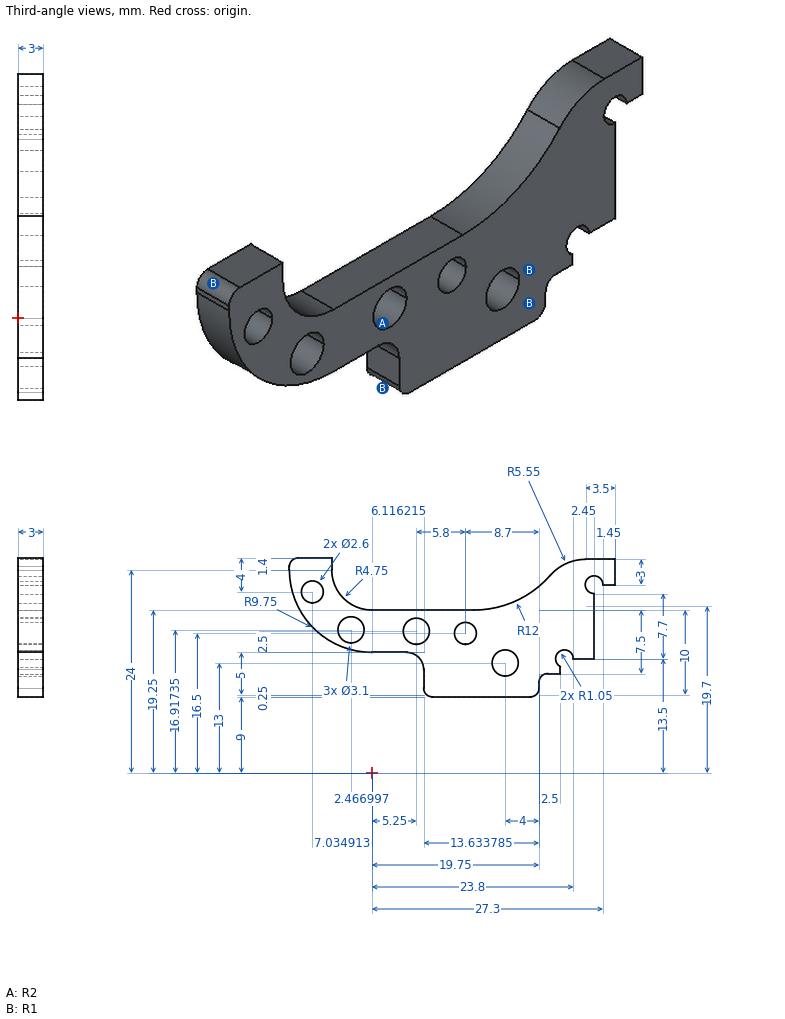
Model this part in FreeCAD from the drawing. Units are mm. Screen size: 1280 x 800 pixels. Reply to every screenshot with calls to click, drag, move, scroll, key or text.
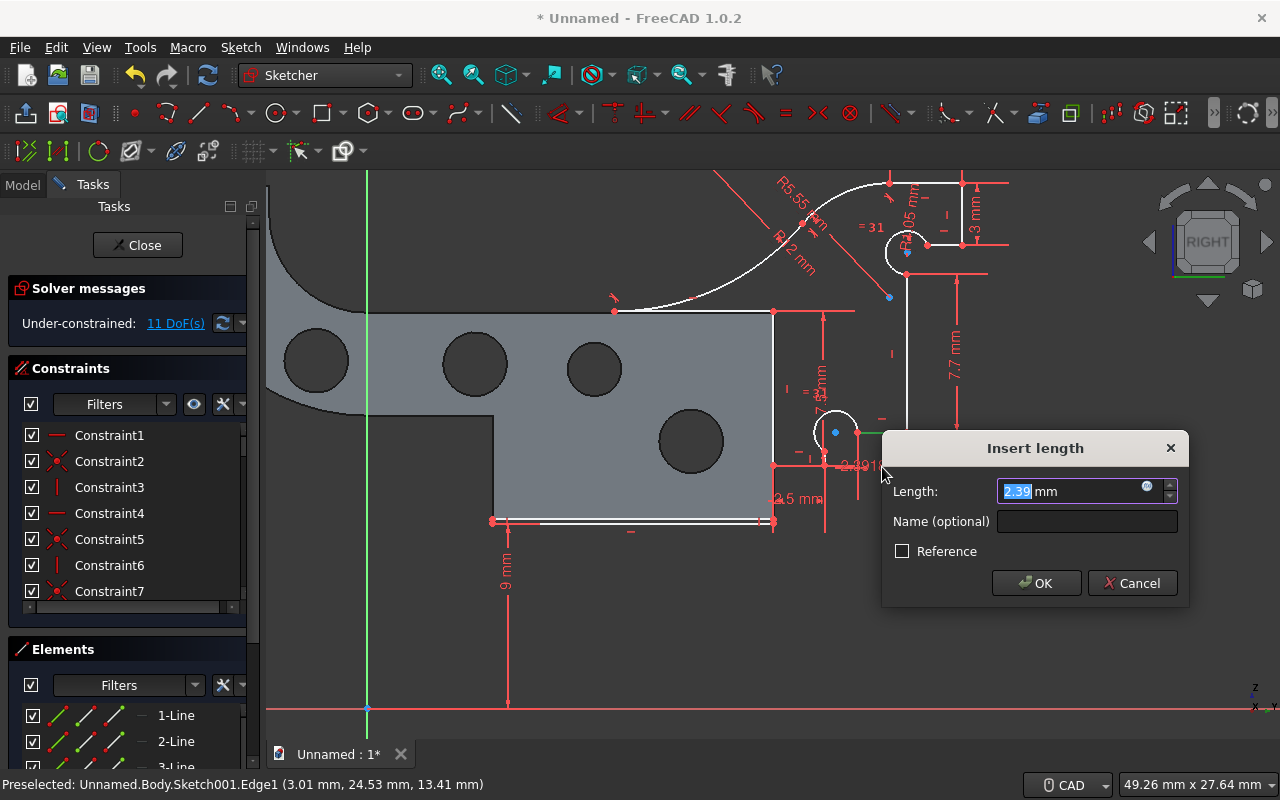
text(2.45)
key(Return)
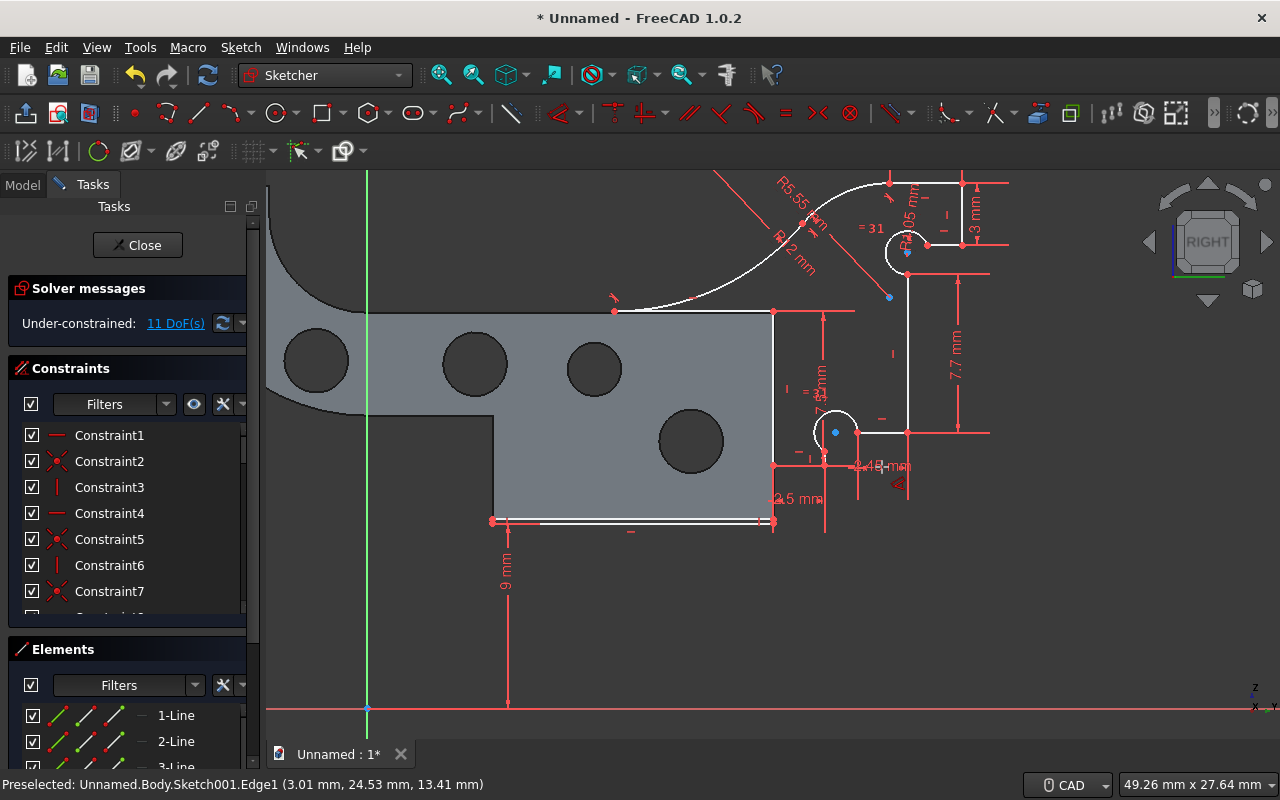
scroll(938, 245, up, 2)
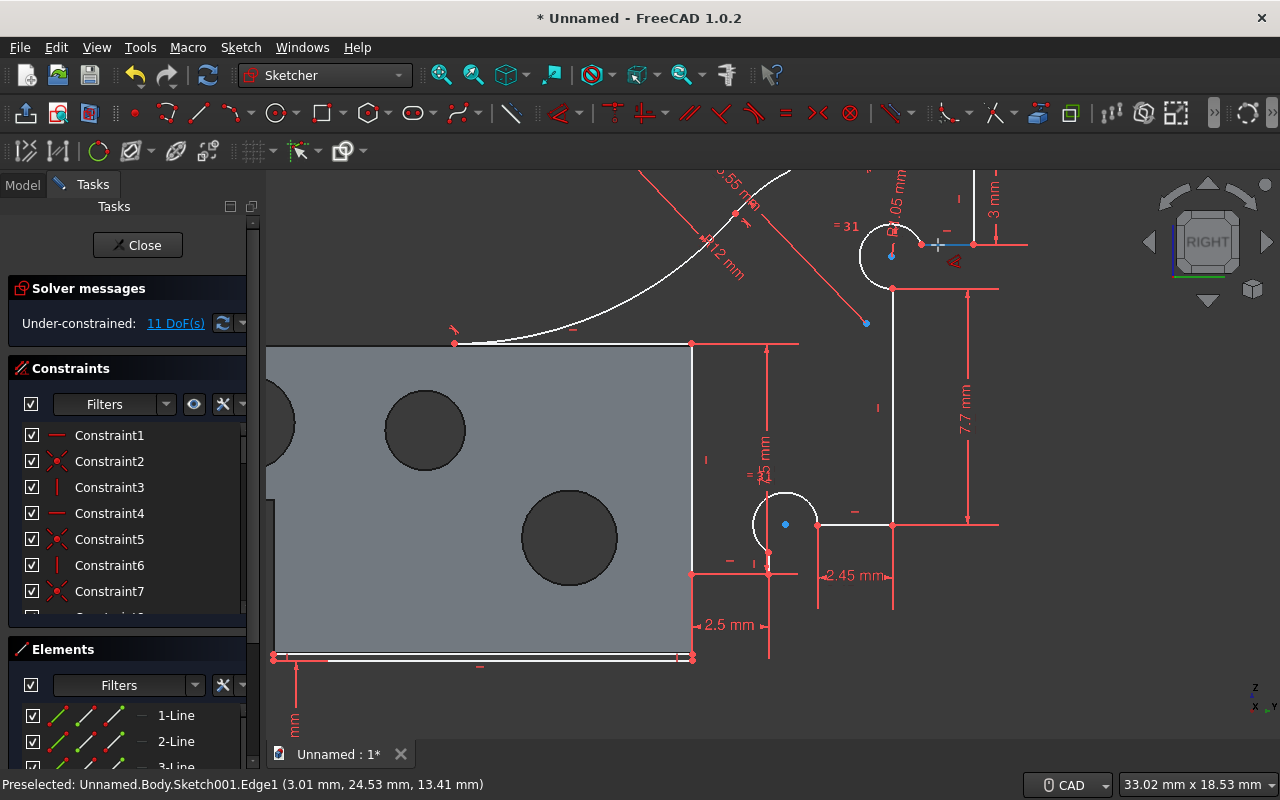
click(937, 245)
click(948, 279)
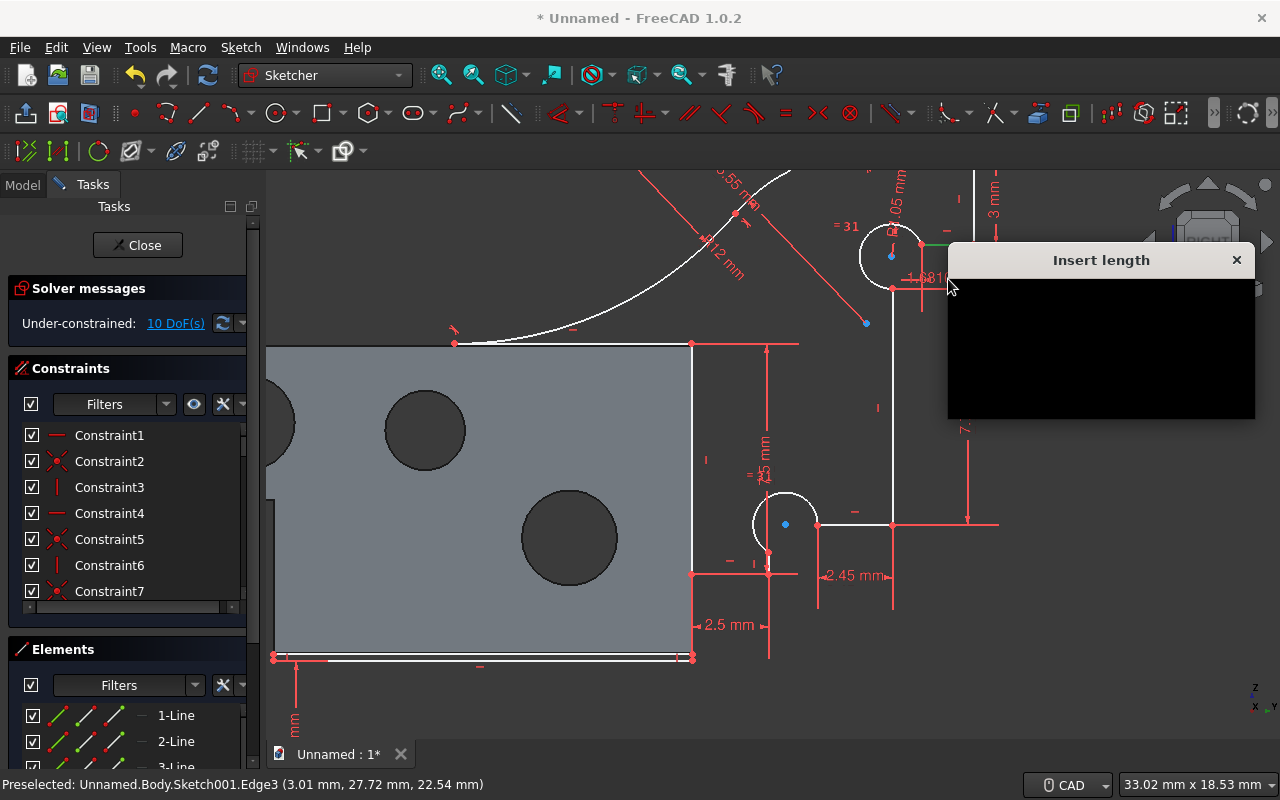
text(1.45)
key(Return)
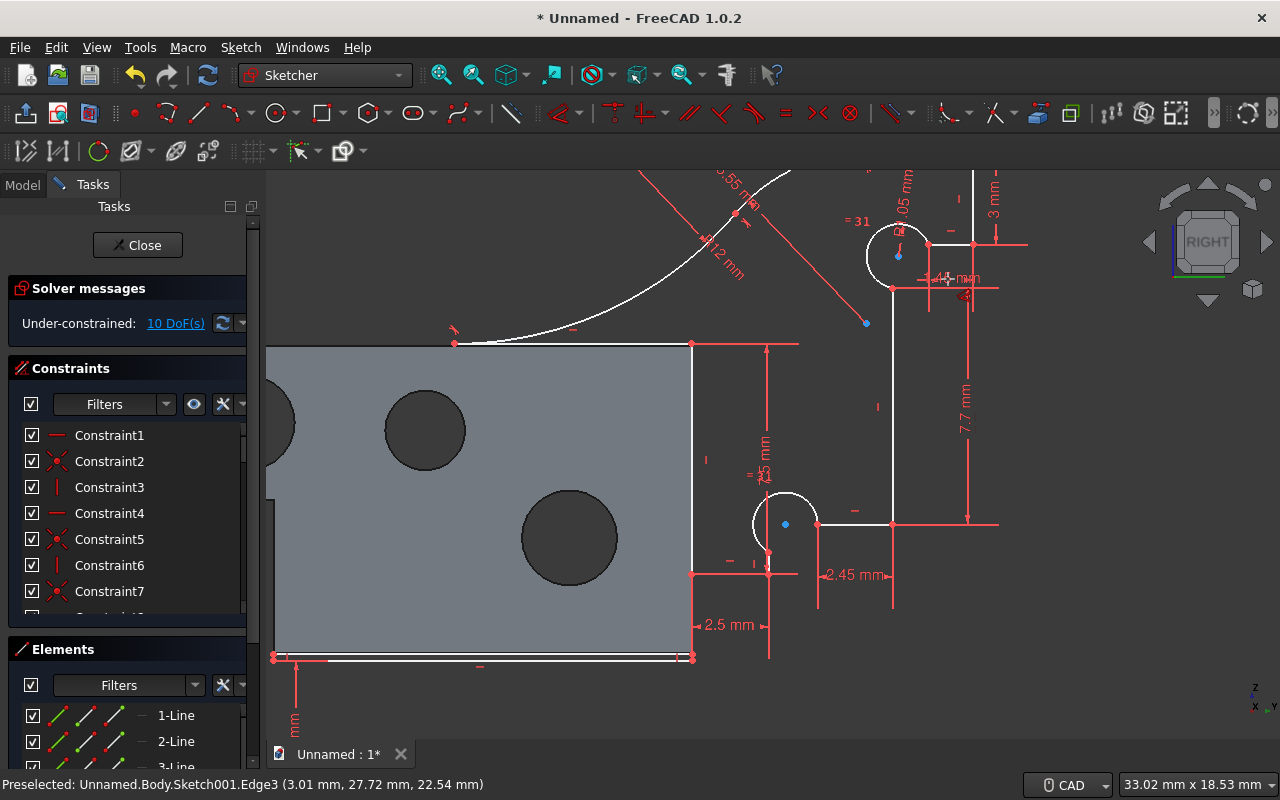
scroll(849, 377, down, 4)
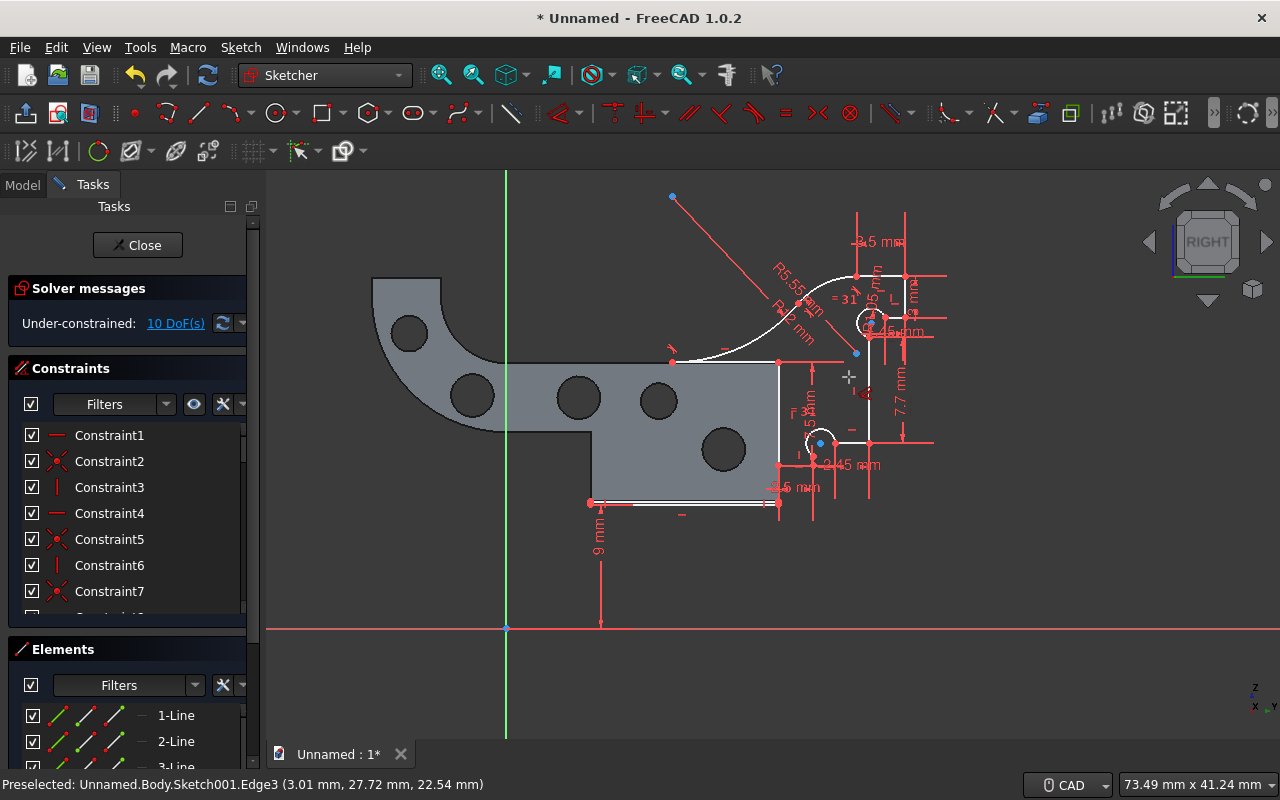
scroll(591, 503, up, 13)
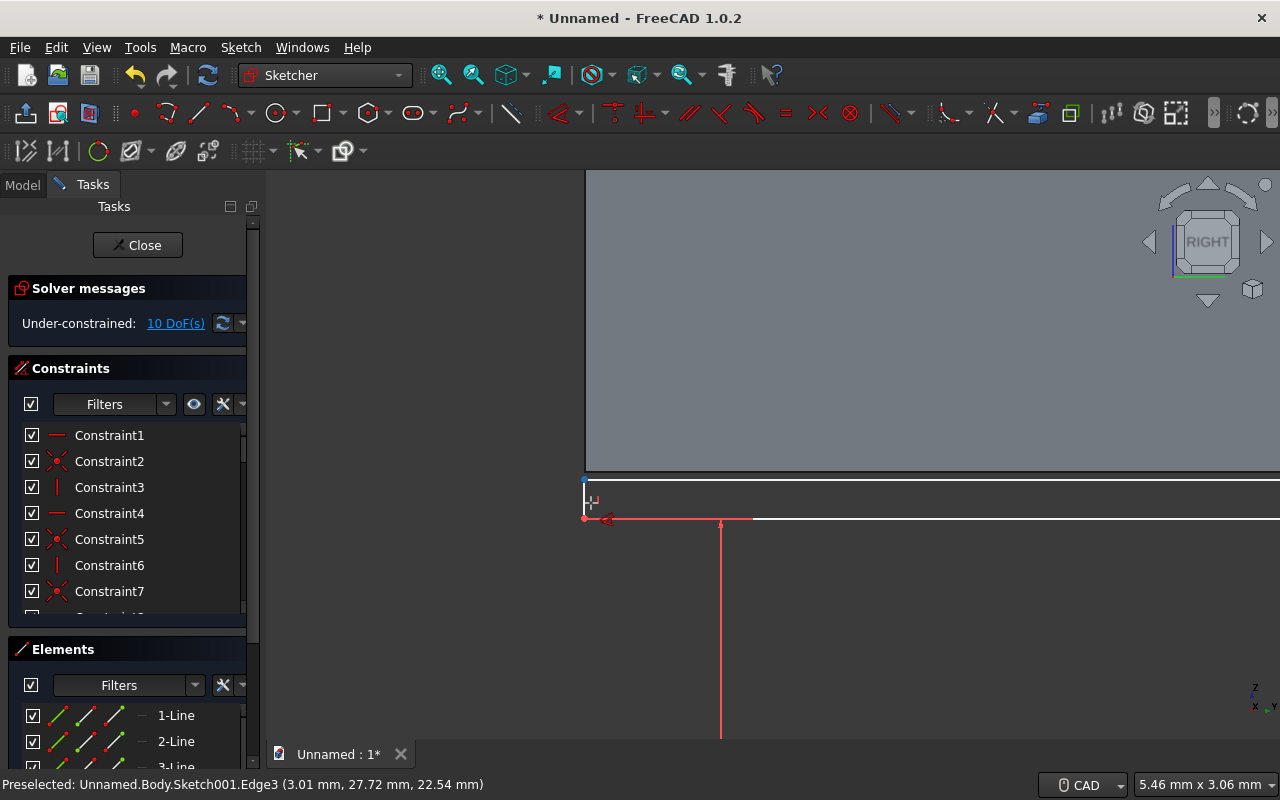
click(584, 499)
click(550, 499)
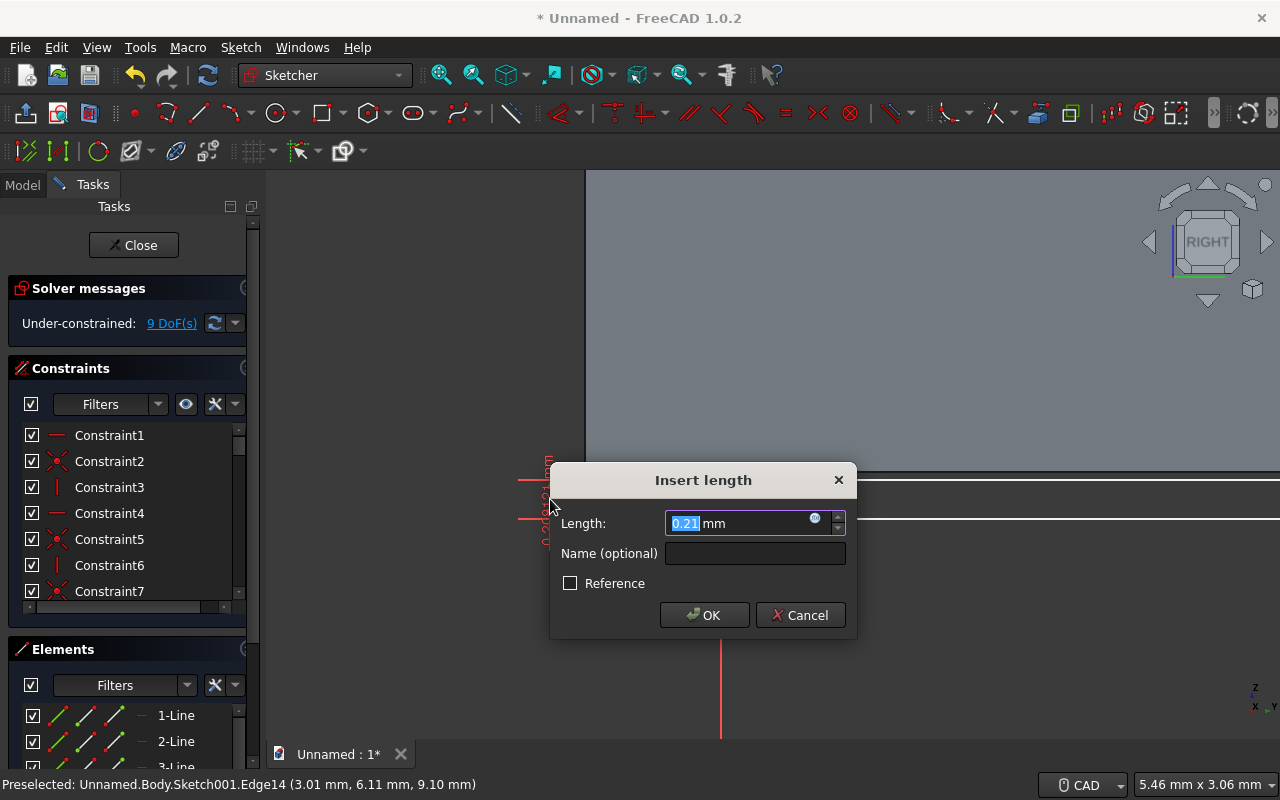
text(0.25)
key(Return)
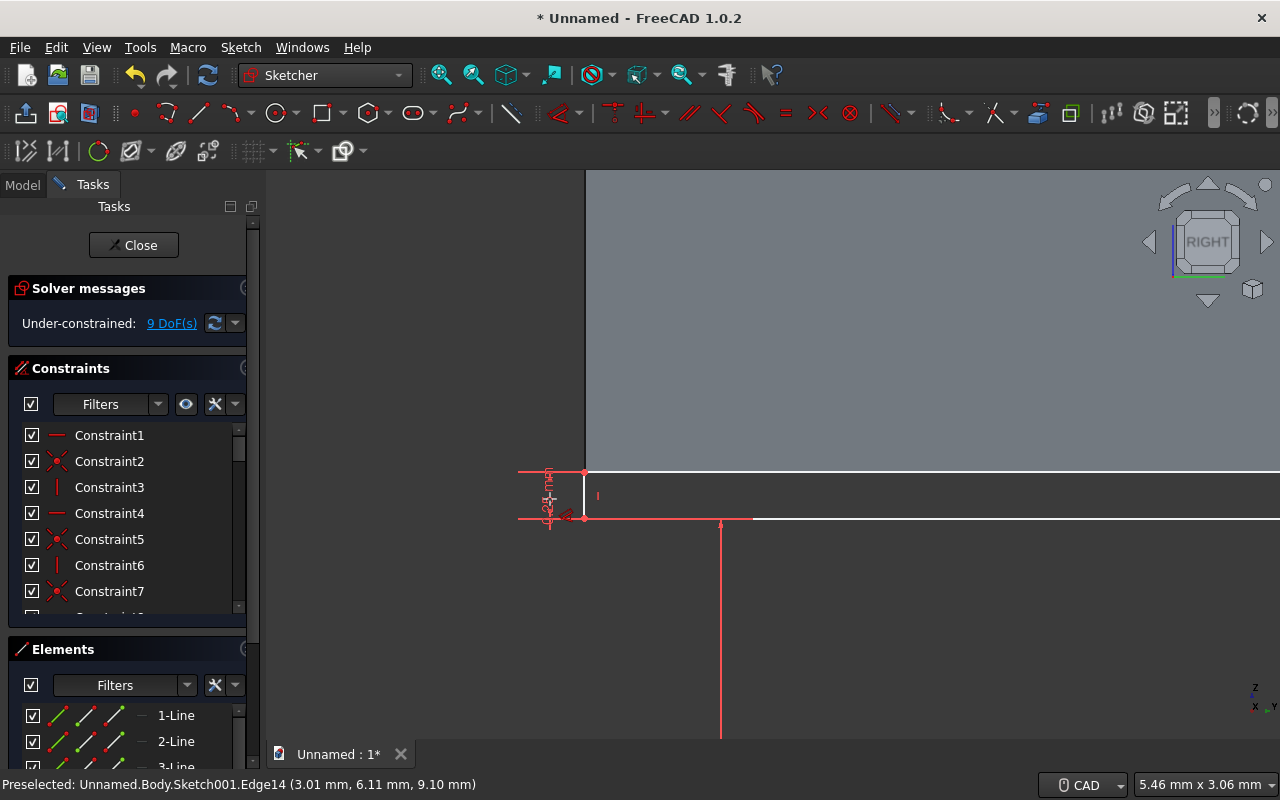
scroll(591, 503, down, 13)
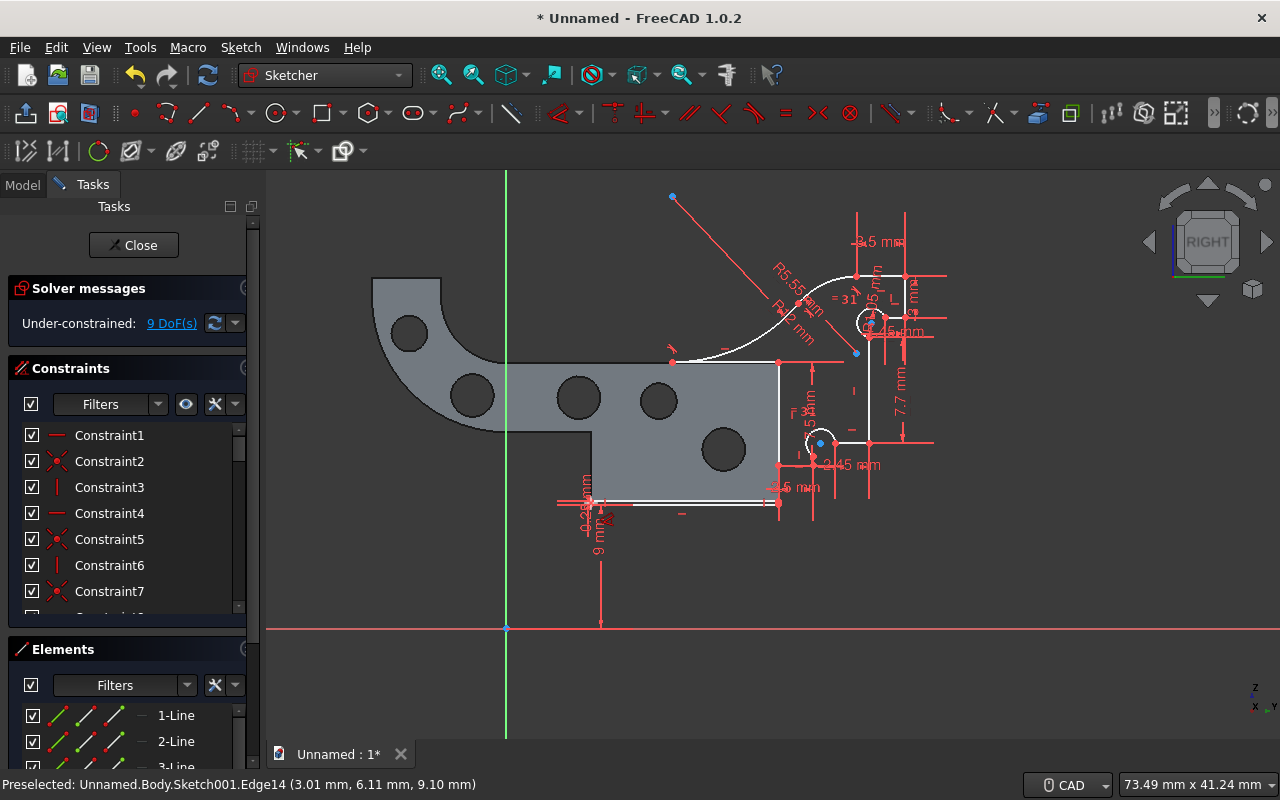
click(835, 443)
click(671, 663)